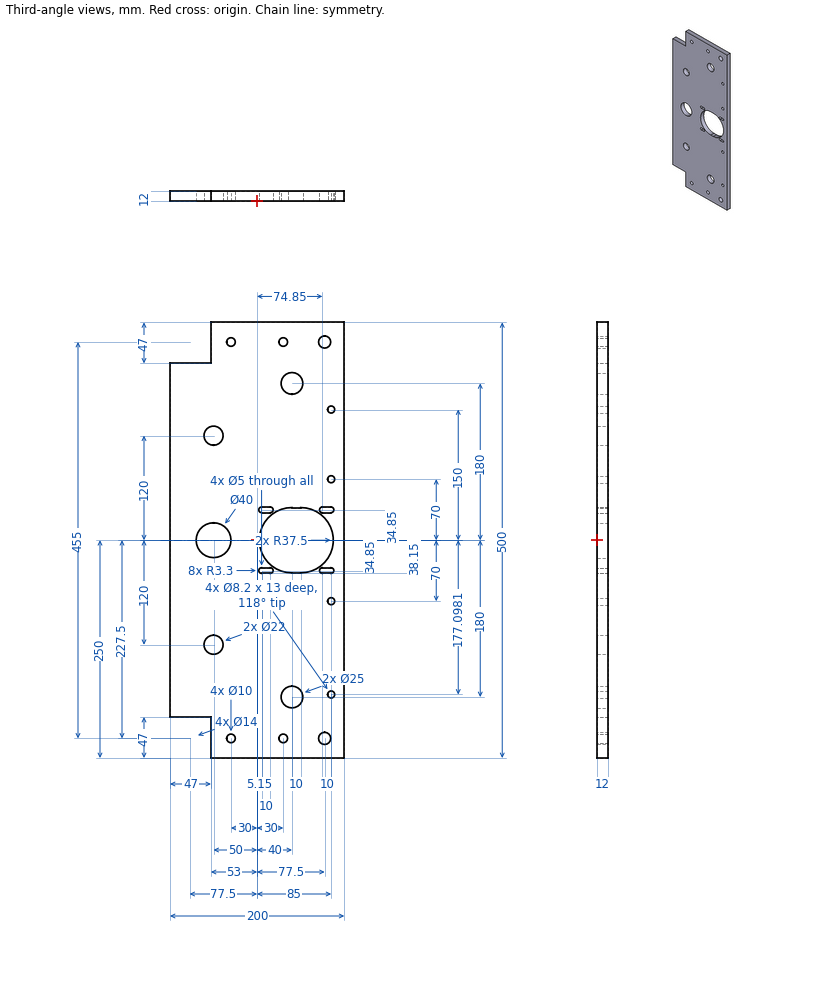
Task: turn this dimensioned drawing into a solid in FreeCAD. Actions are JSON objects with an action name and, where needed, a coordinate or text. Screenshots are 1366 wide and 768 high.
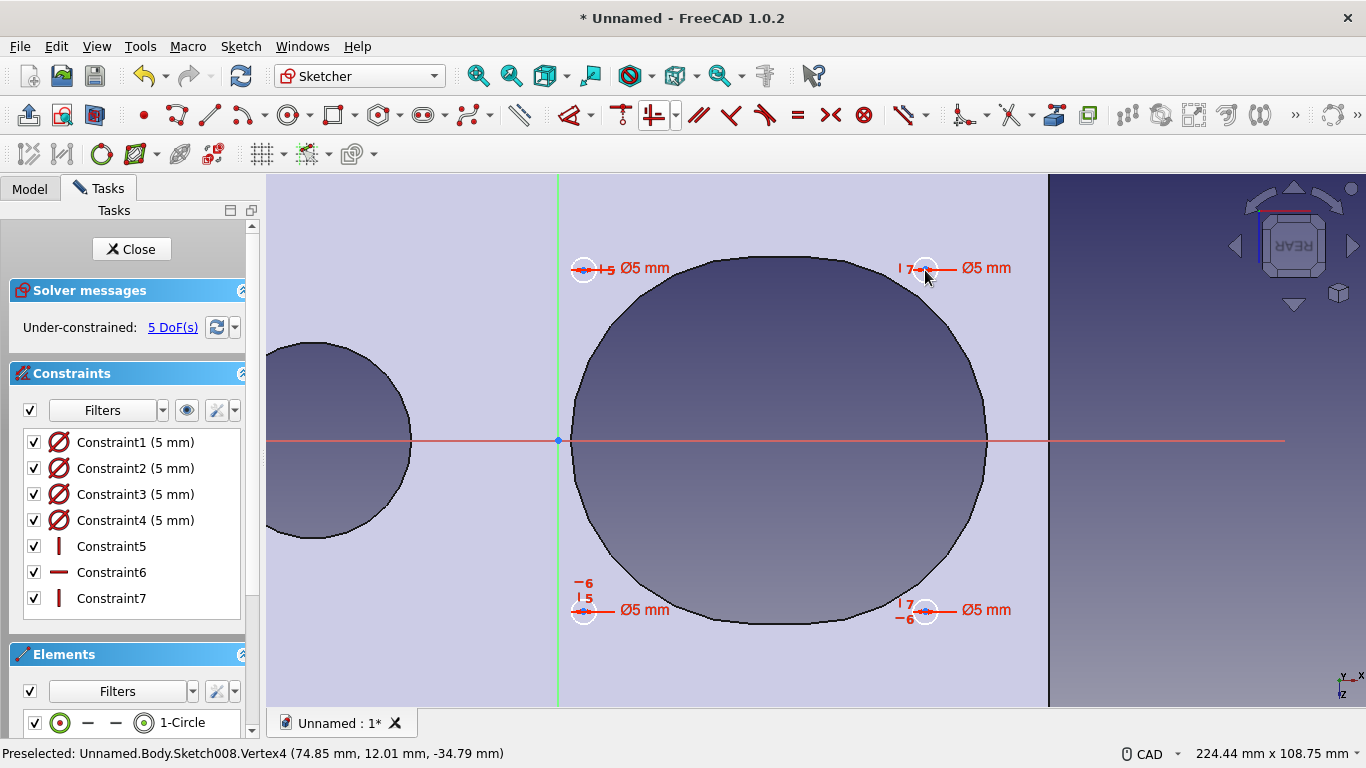
{"action": "left_click", "coordinate": [584, 270]}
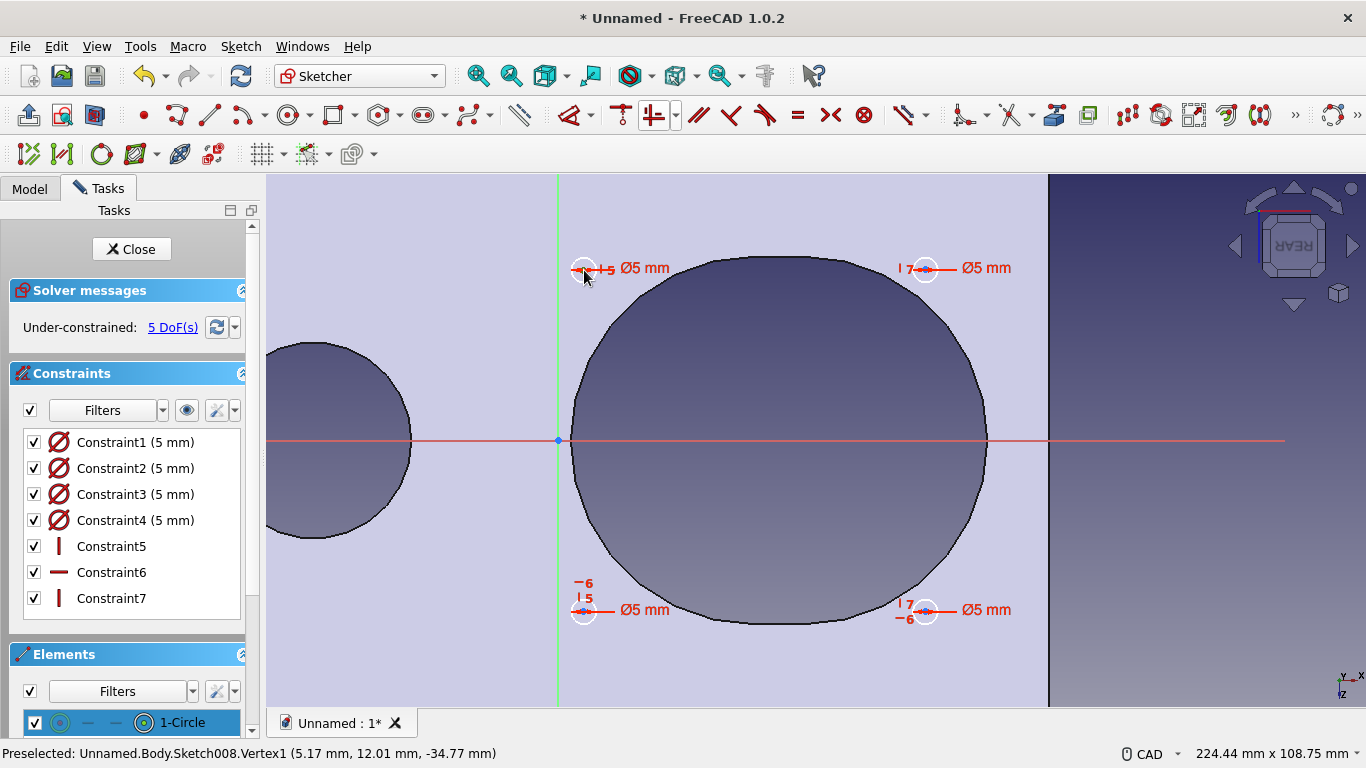
{"action": "left_click", "coordinate": [925, 270]}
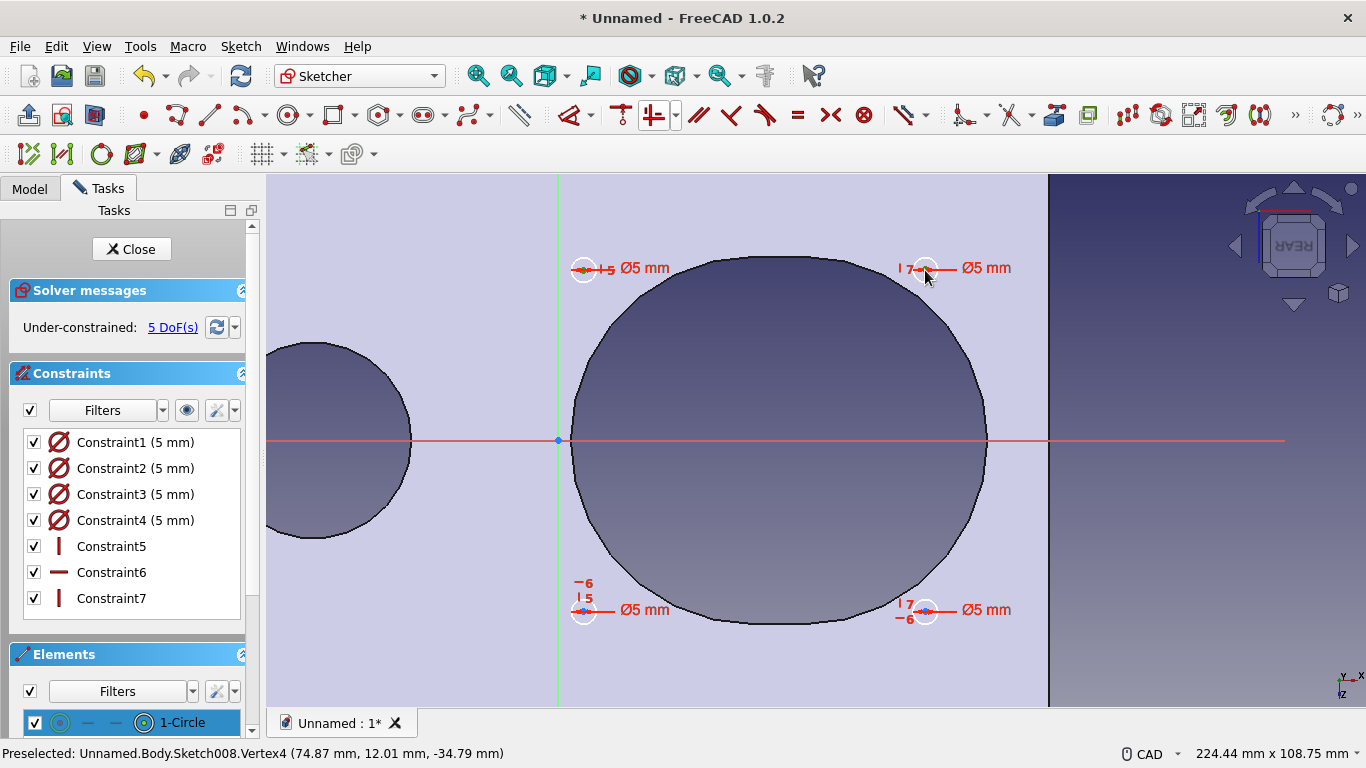
{"action": "key", "text": "h"}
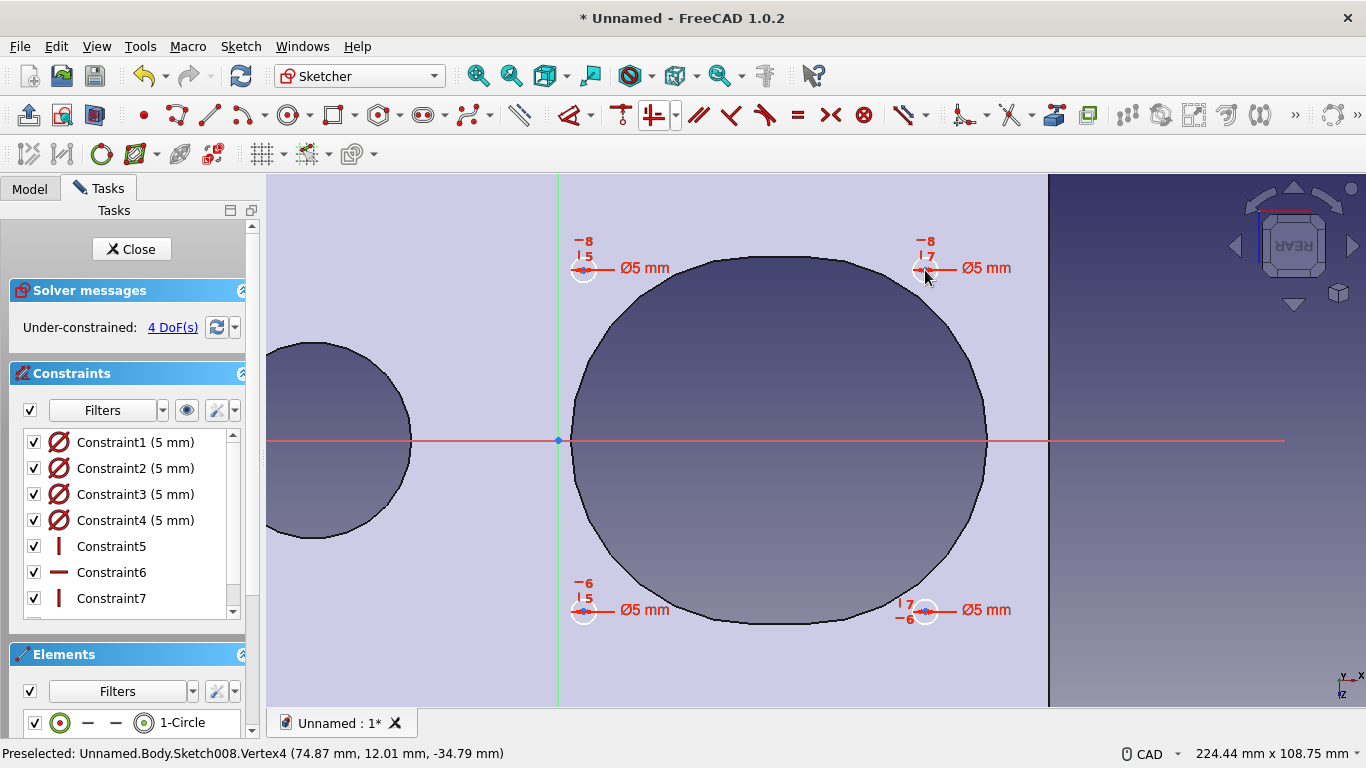
{"action": "key", "text": "d"}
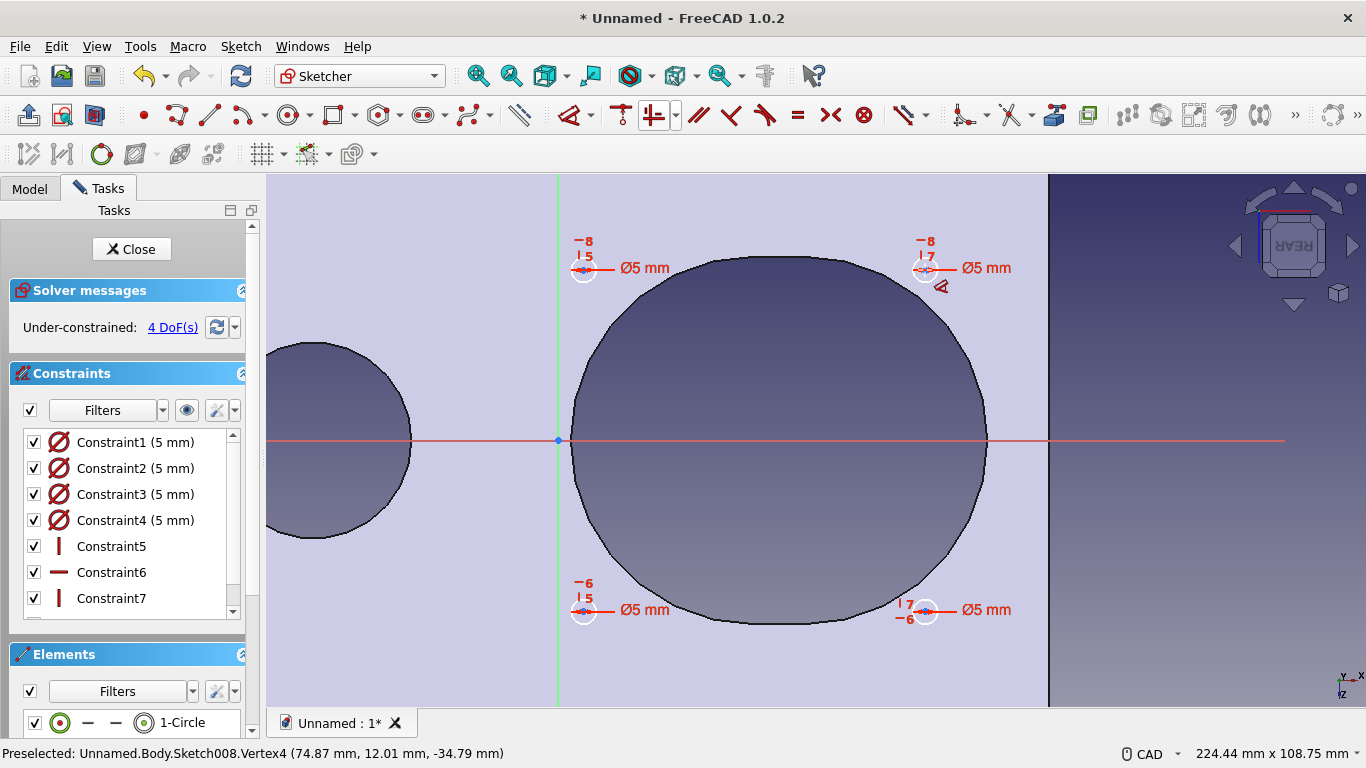
{"action": "scroll", "coordinate": [584, 270], "scroll_direction": "up", "scroll_amount": 3}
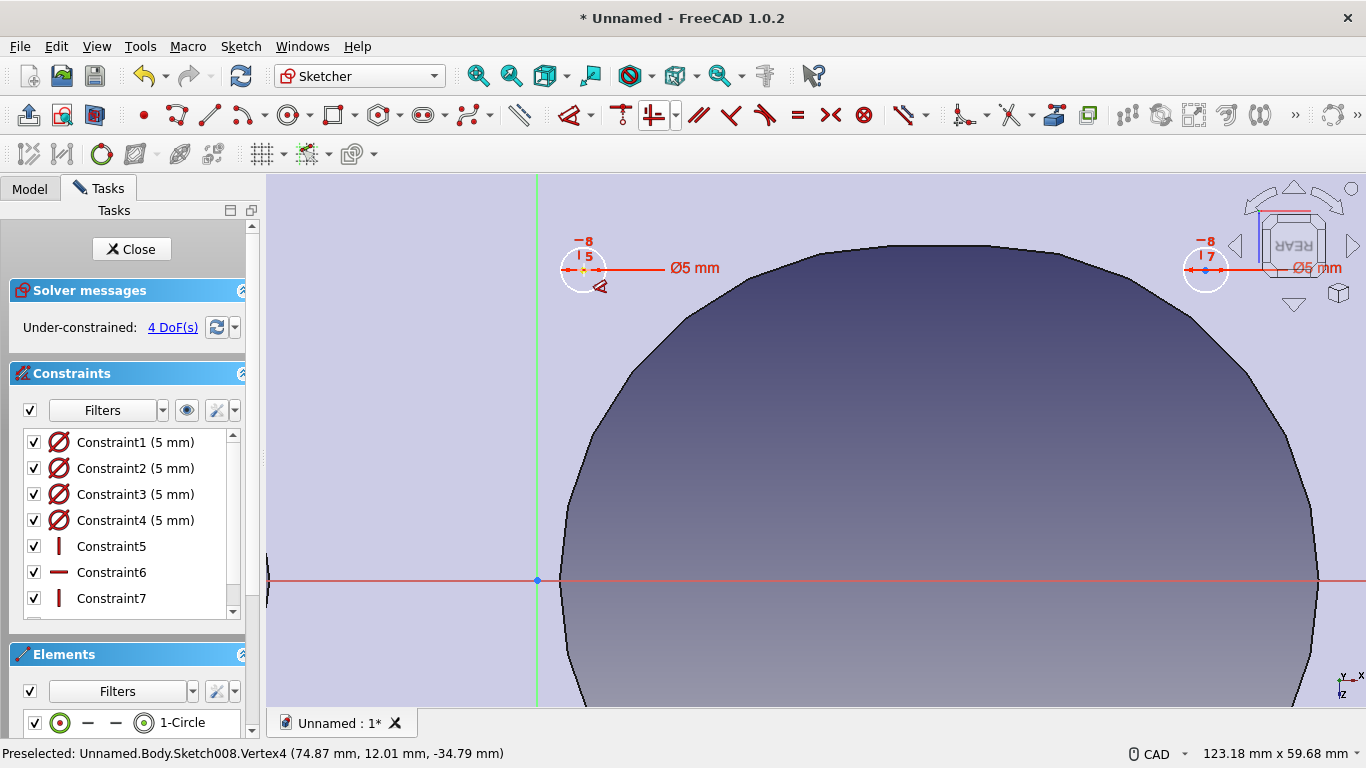
{"action": "left_click", "coordinate": [583, 270]}
{"action": "left_click", "coordinate": [560, 236]}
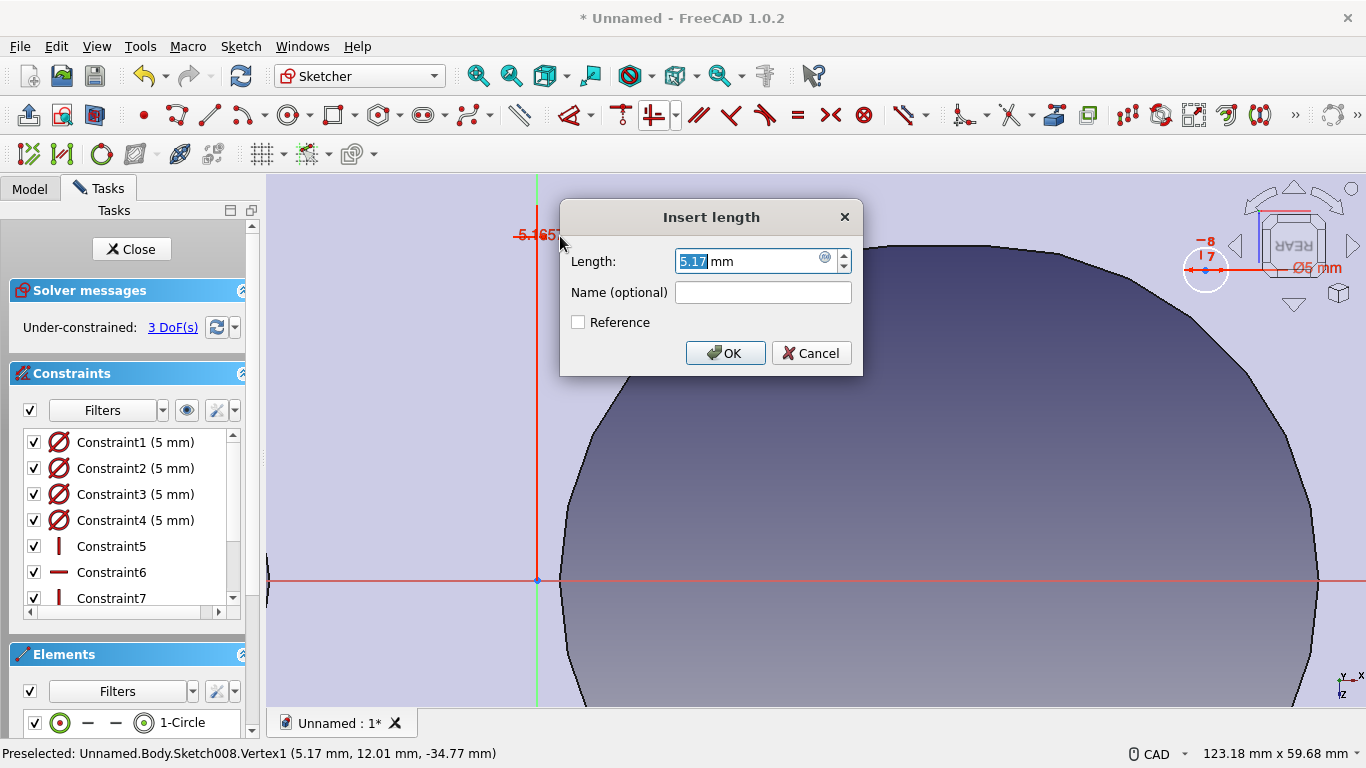
{"action": "type", "text": "5.15"}
{"action": "key", "text": "Return"}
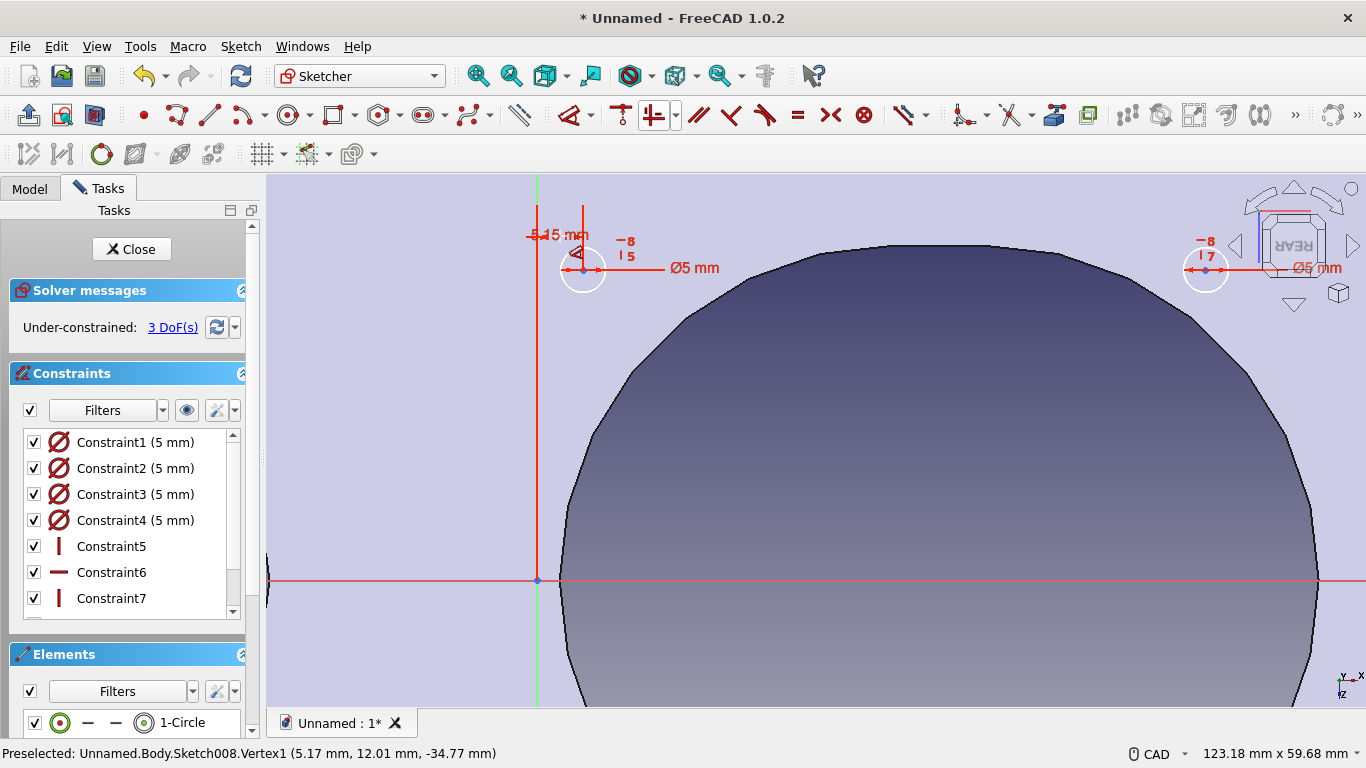
{"action": "left_click", "coordinate": [583, 270]}
{"action": "left_click", "coordinate": [503, 425]}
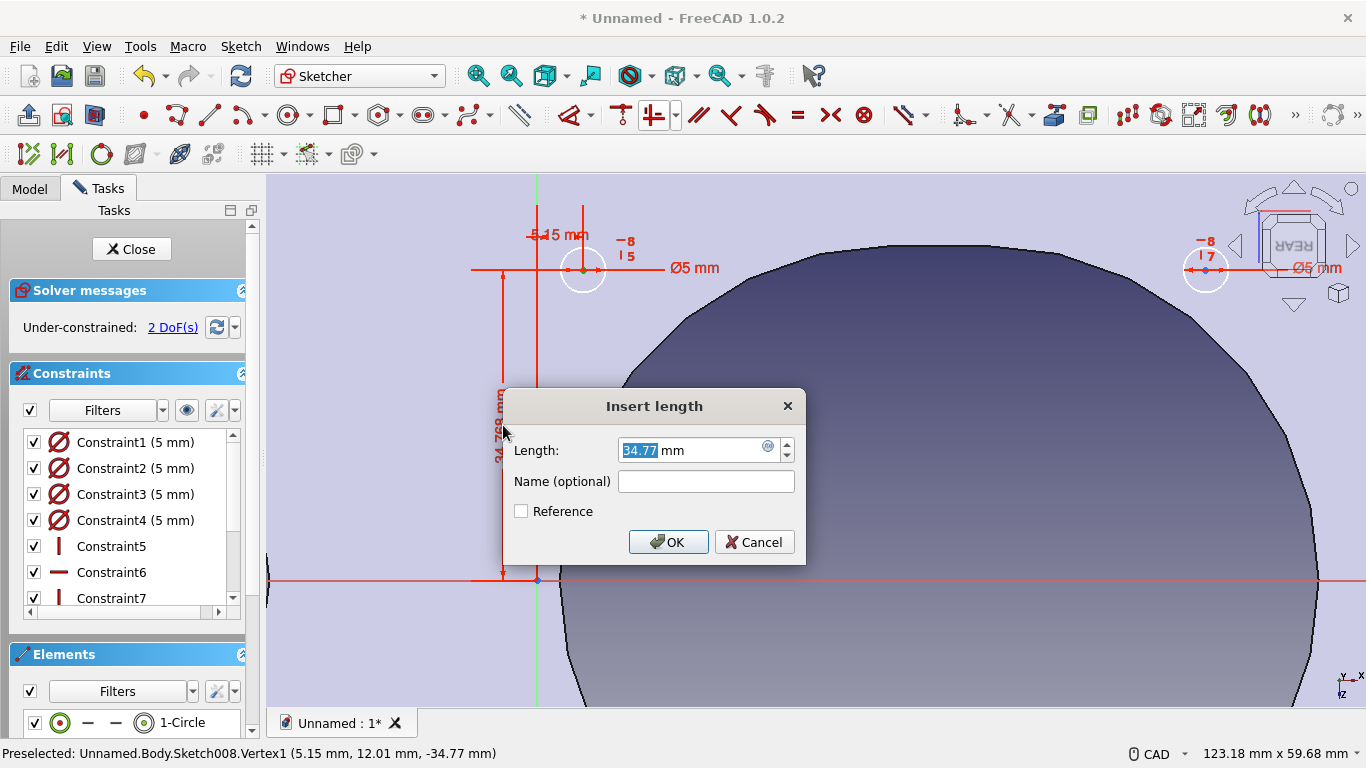
{"action": "type", "text": "34.85"}
{"action": "key", "text": "Return"}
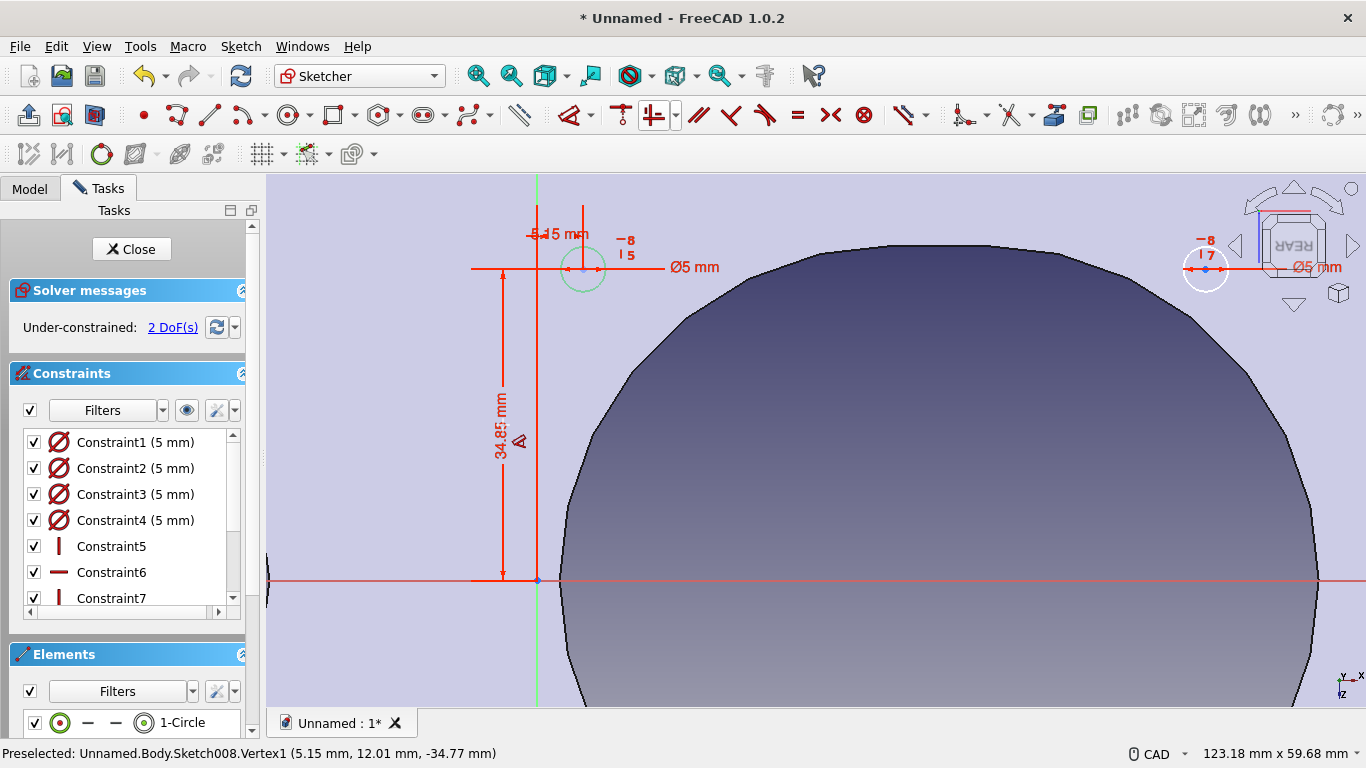
{"action": "scroll", "coordinate": [583, 270], "scroll_direction": "down", "scroll_amount": 3}